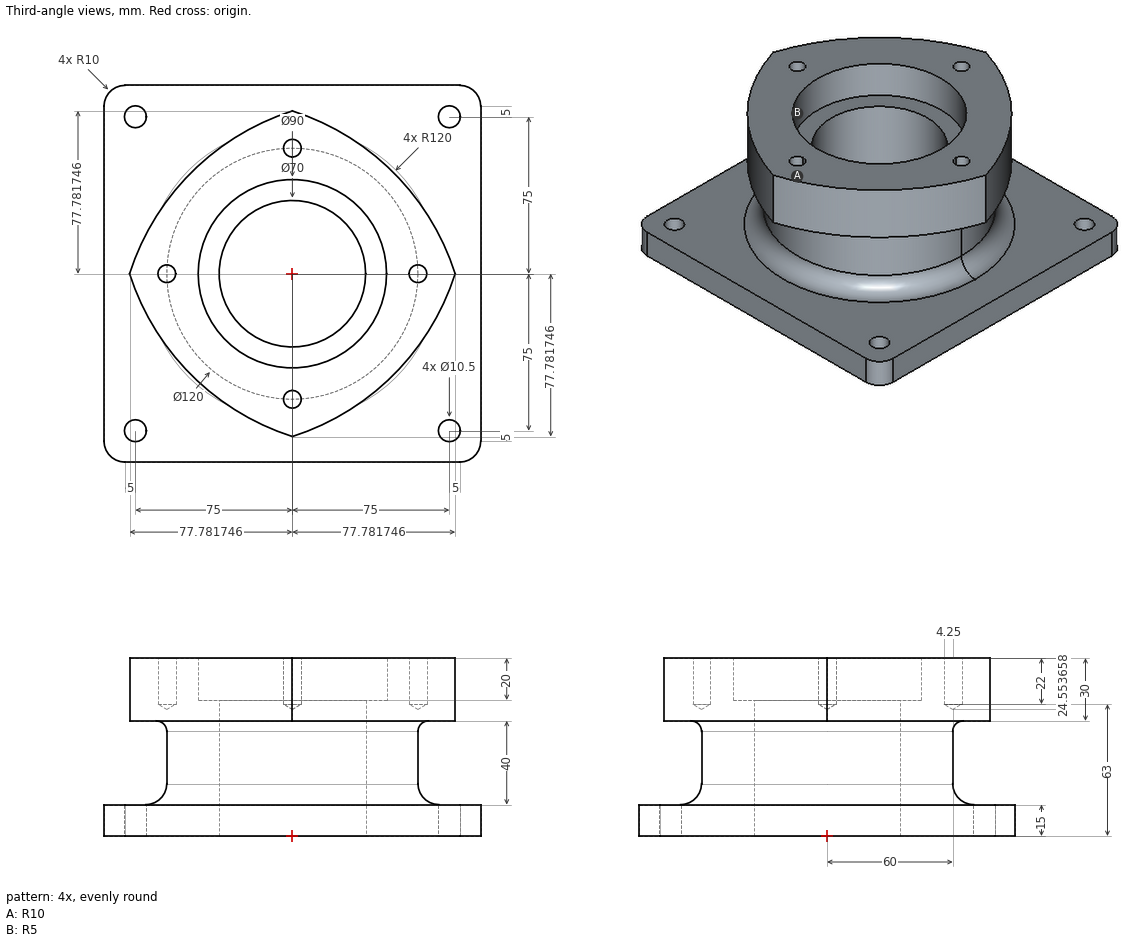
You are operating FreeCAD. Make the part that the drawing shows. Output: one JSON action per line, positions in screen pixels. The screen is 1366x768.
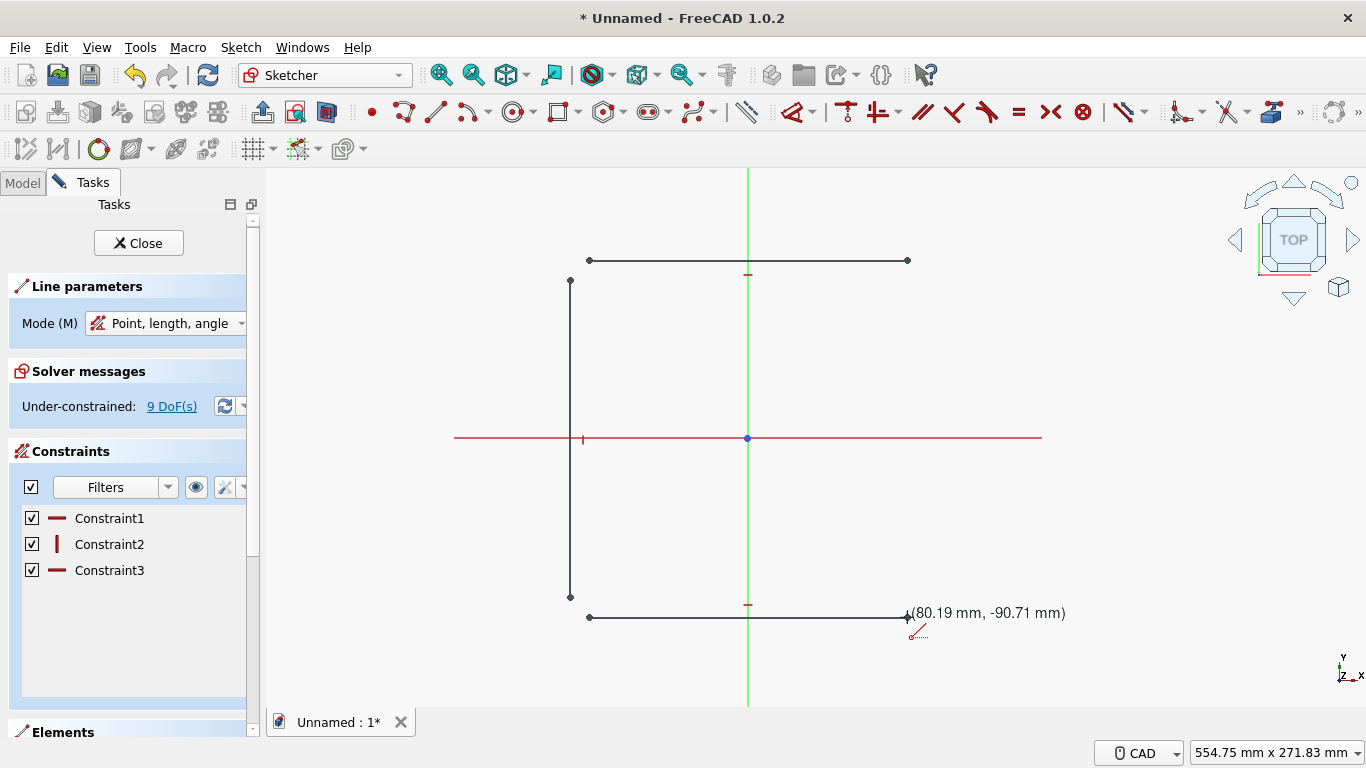
{"action": "left_click", "coordinate": [926, 597]}
{"action": "left_click", "coordinate": [926, 280]}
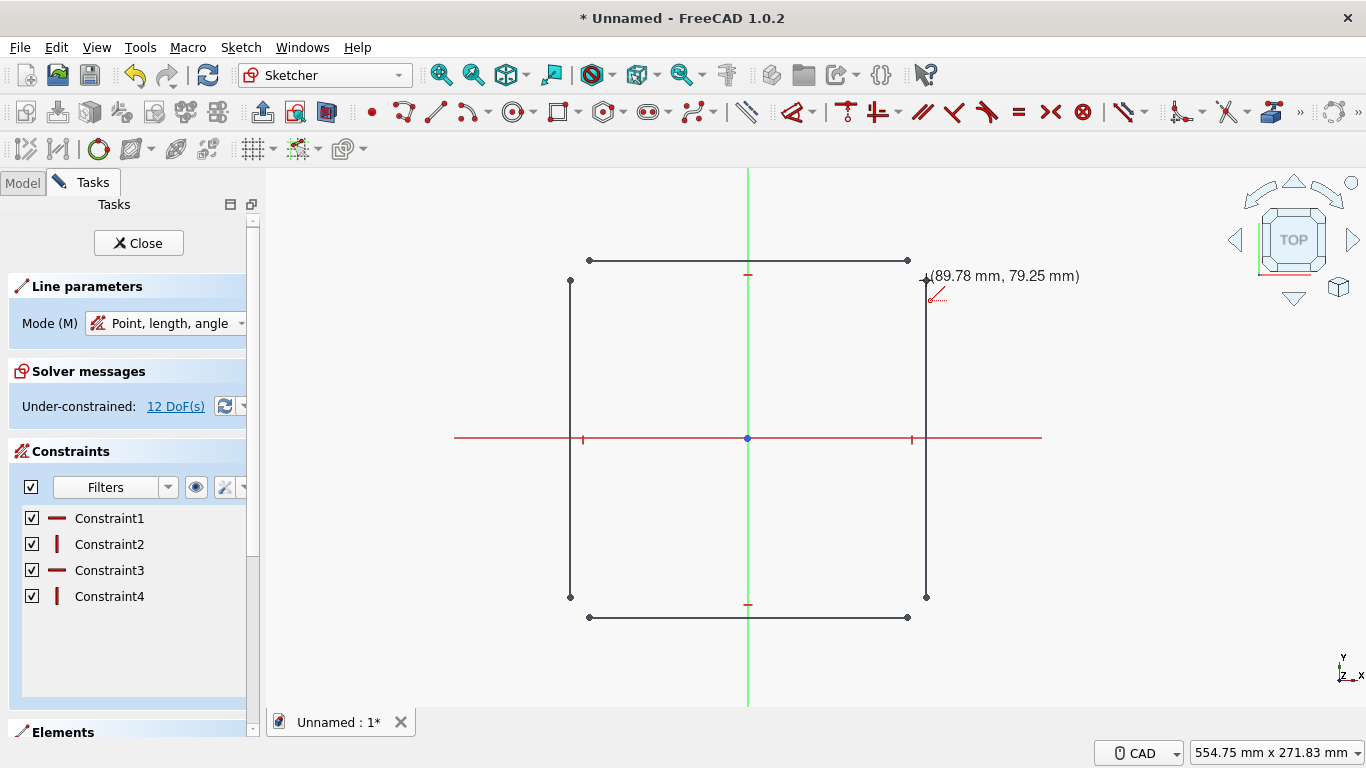
{"action": "left_click", "coordinate": [490, 112]}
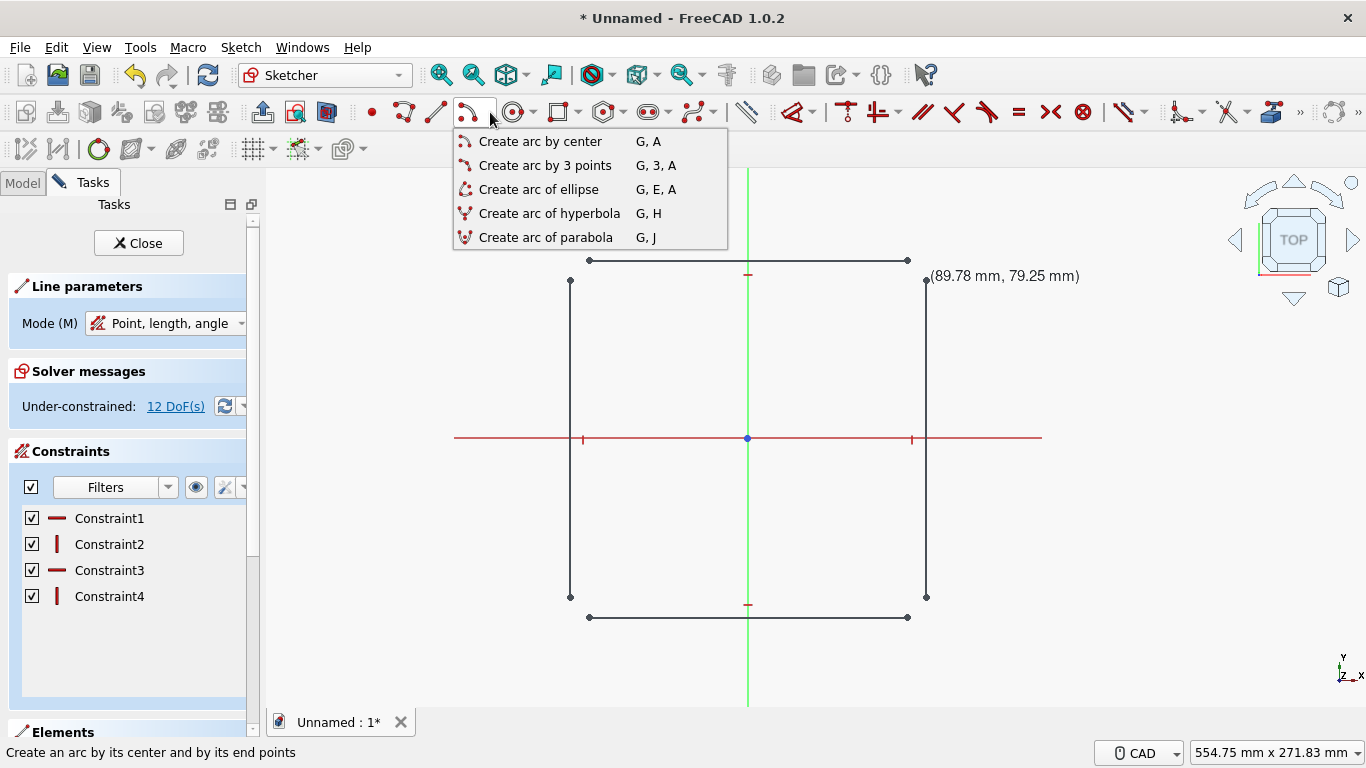
{"action": "left_click", "coordinate": [590, 165]}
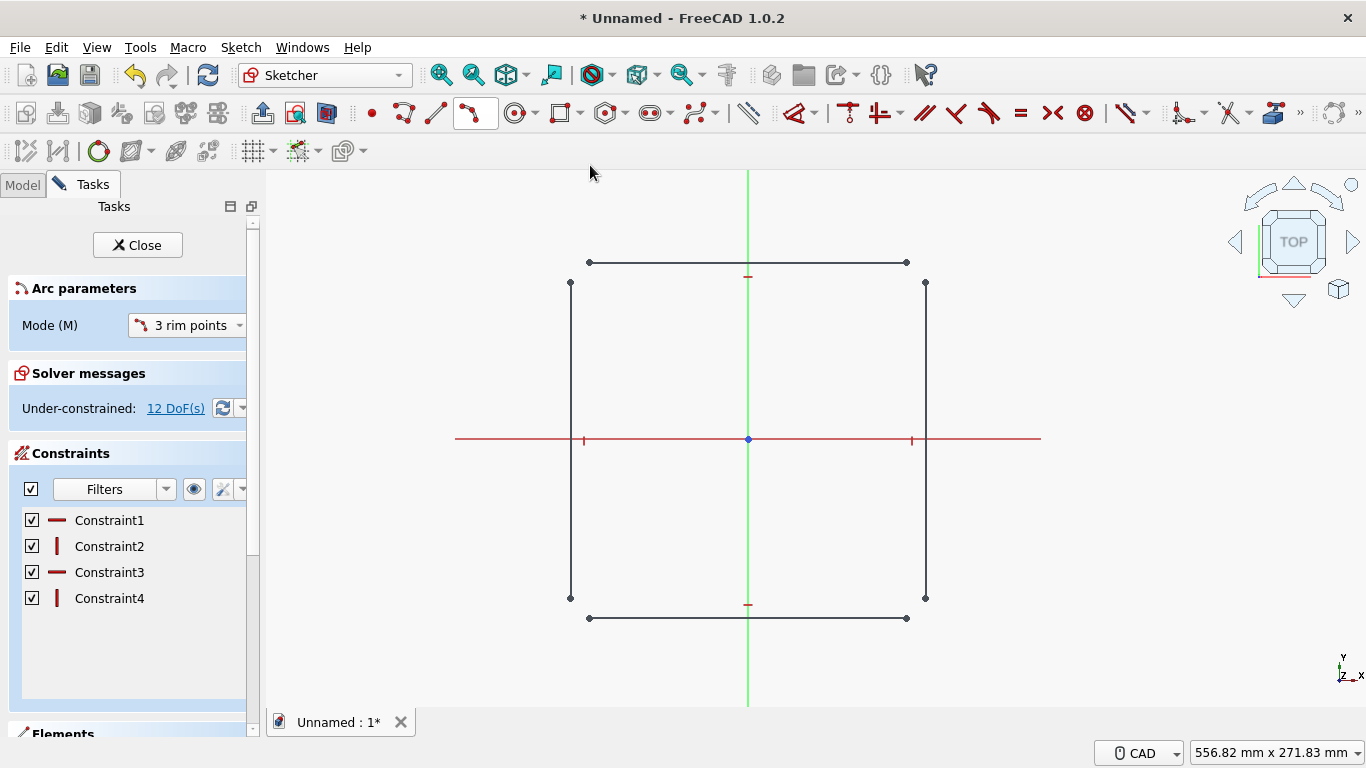
{"action": "left_click", "coordinate": [590, 263]}
{"action": "left_click", "coordinate": [571, 283]}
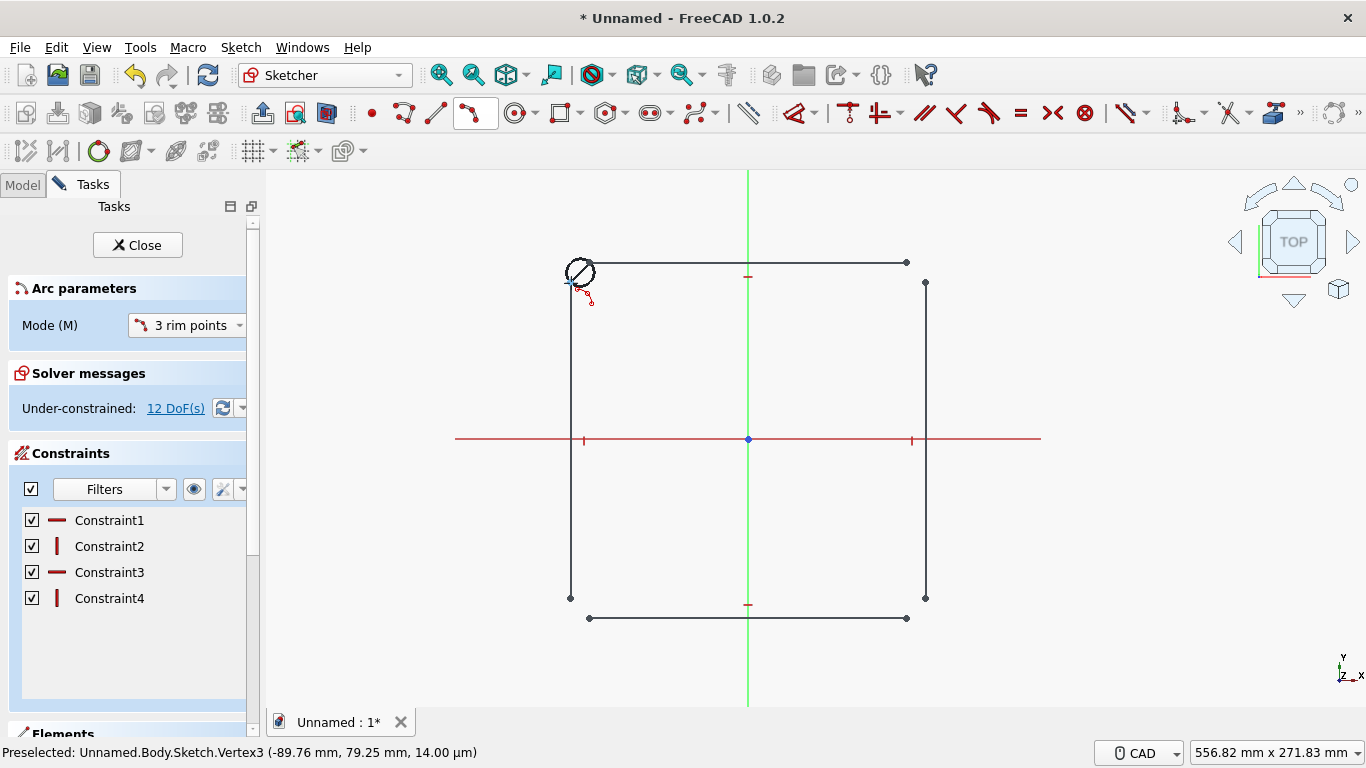
{"action": "scroll", "coordinate": [576, 267], "scroll_direction": "up", "scroll_amount": 6}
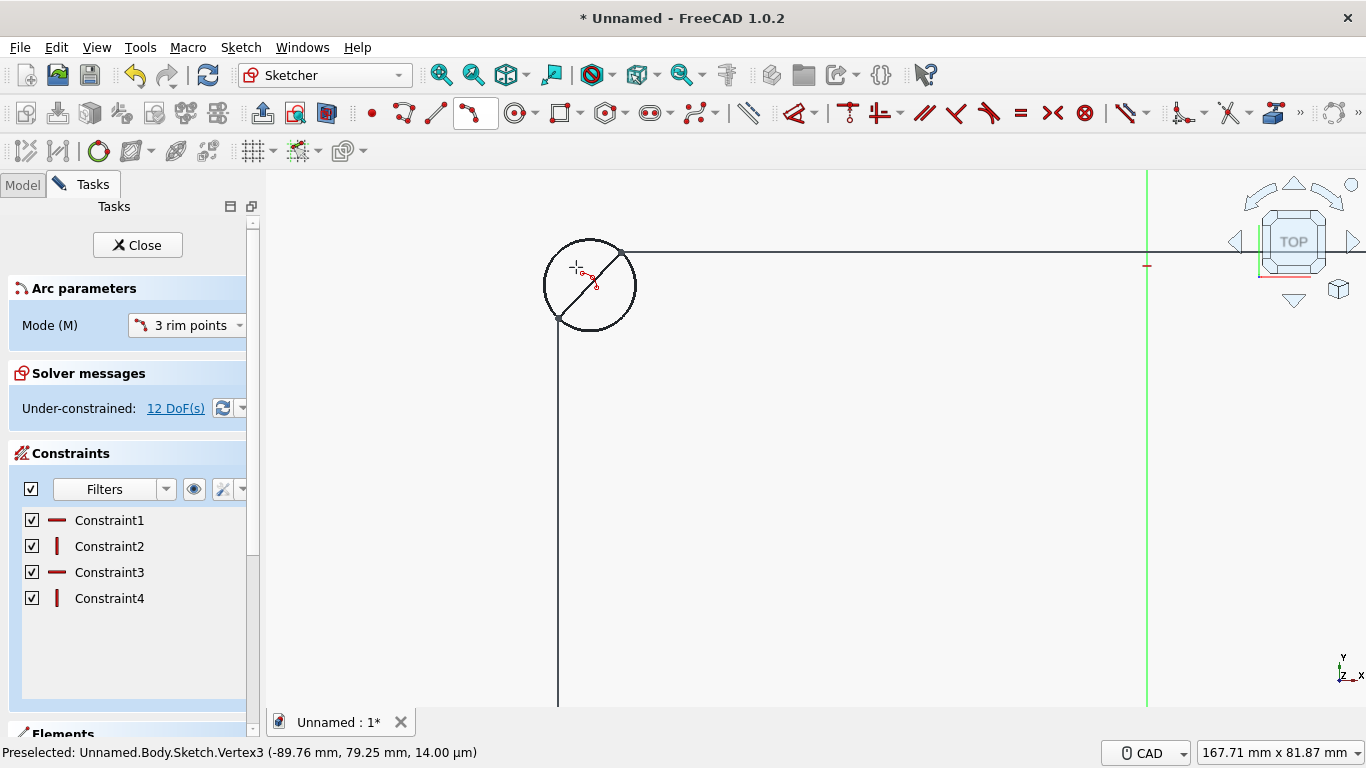
{"action": "left_click", "coordinate": [576, 267]}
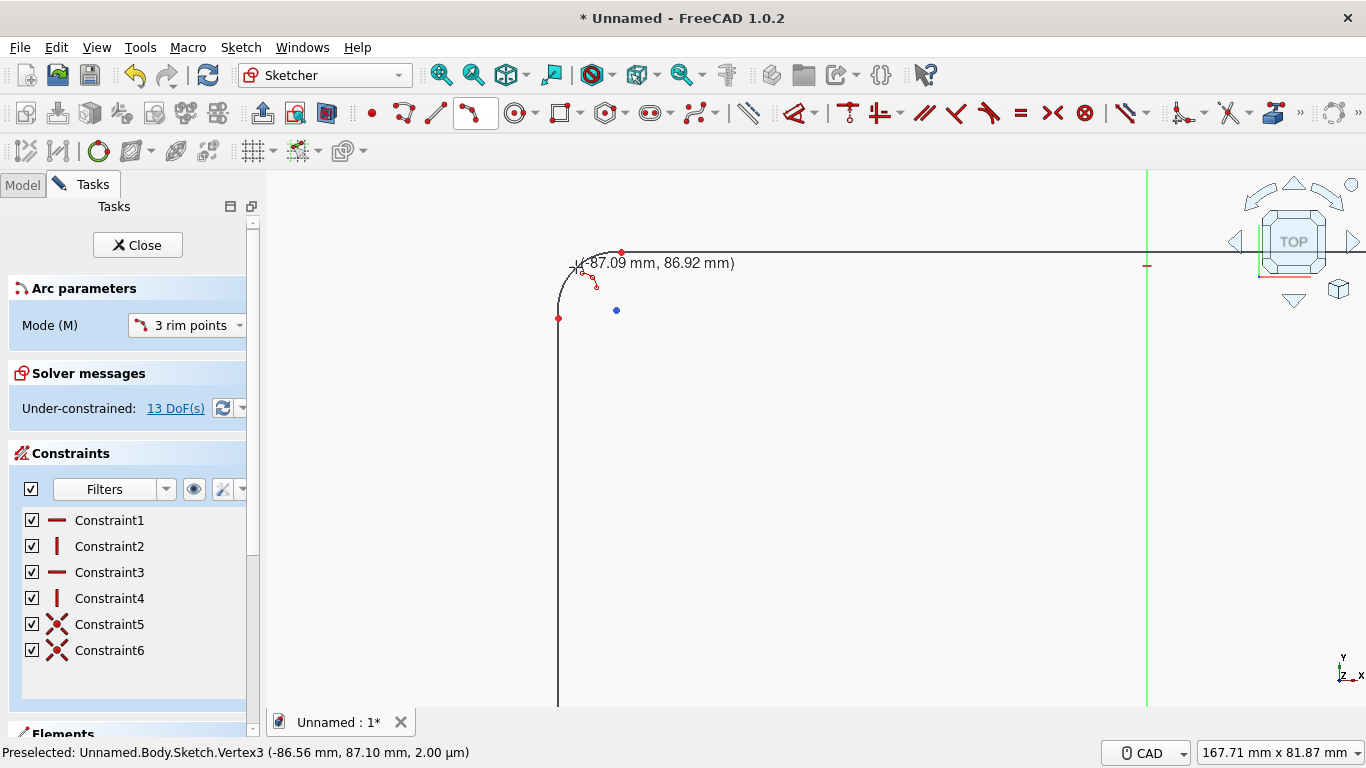
{"action": "scroll", "coordinate": [575, 266], "scroll_direction": "down", "scroll_amount": 6}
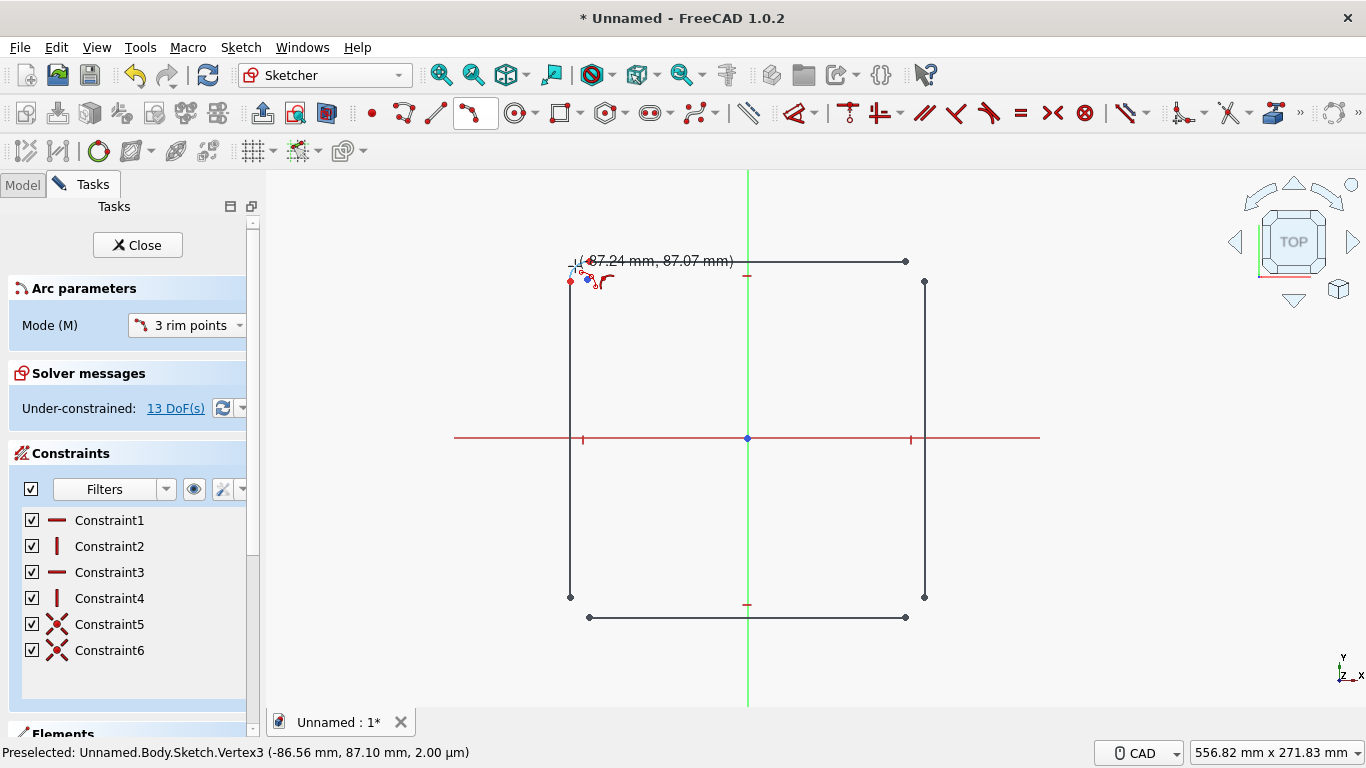
{"action": "left_click", "coordinate": [570, 598]}
{"action": "left_click", "coordinate": [589, 618]}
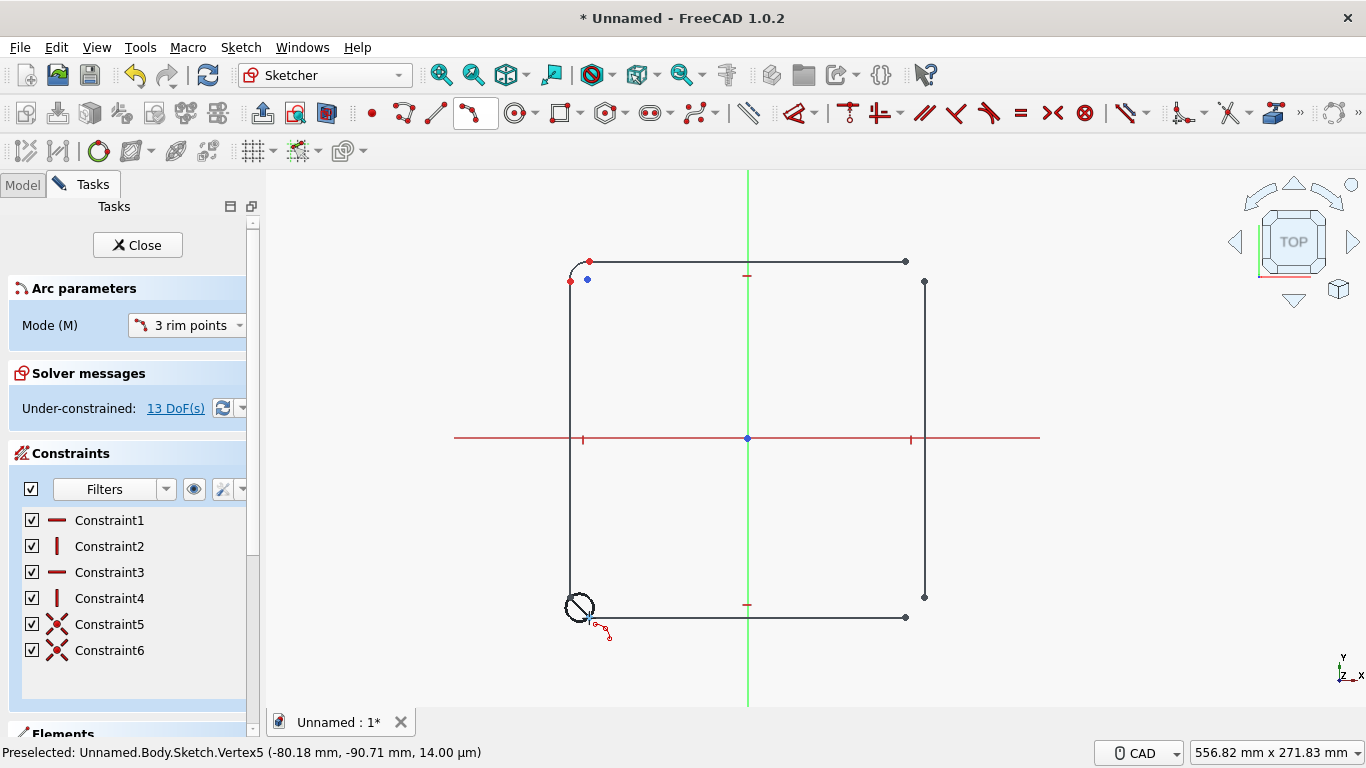
{"action": "scroll", "coordinate": [576, 610], "scroll_direction": "up", "scroll_amount": 6}